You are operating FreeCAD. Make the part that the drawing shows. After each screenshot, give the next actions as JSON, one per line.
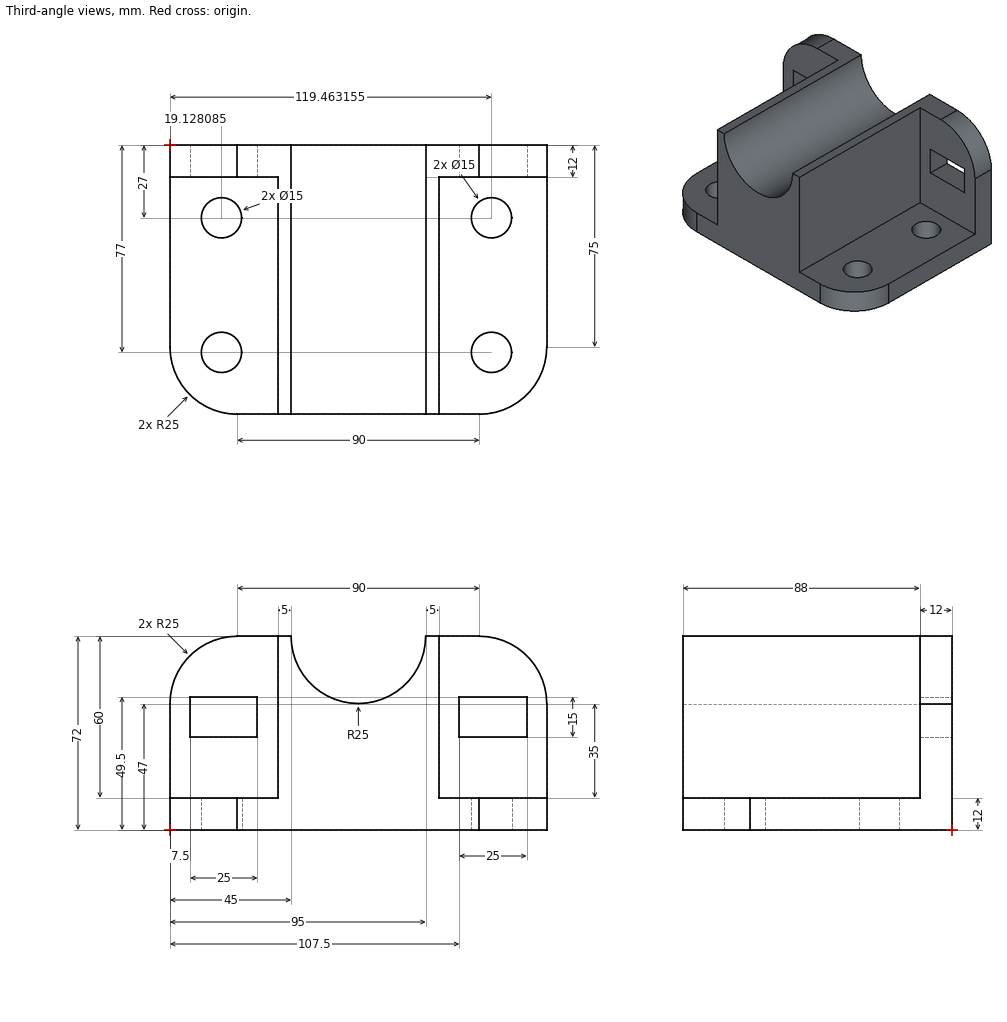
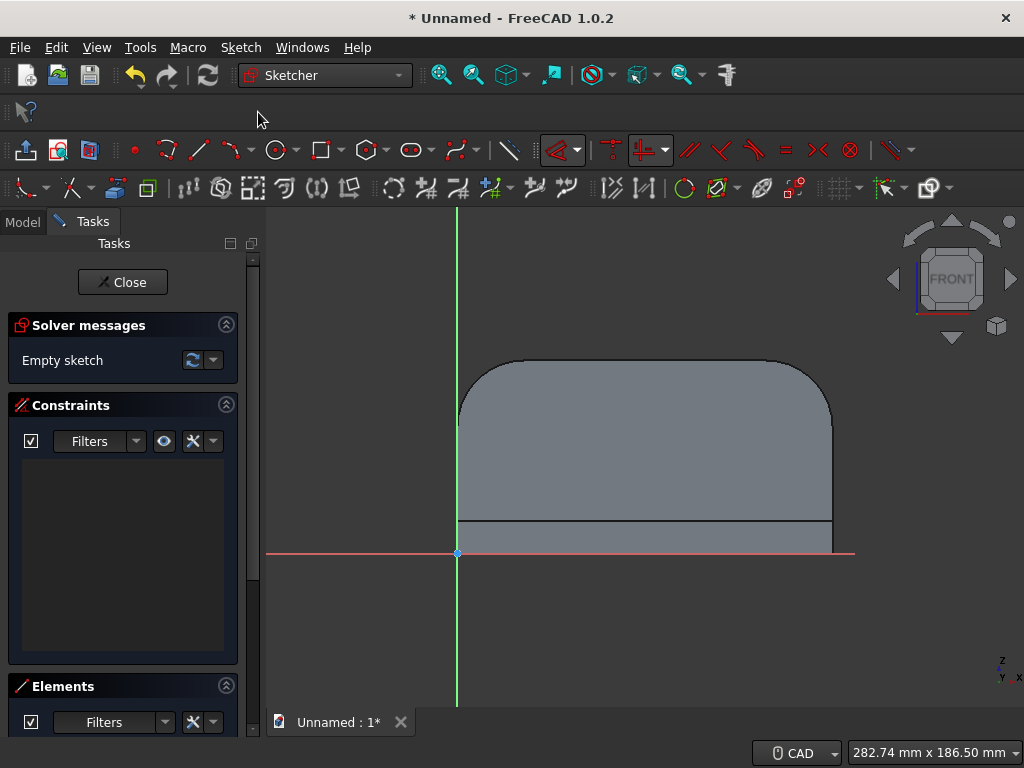
{"action": "scroll", "coordinate": [622, 457], "scroll_direction": "up", "scroll_amount": 2}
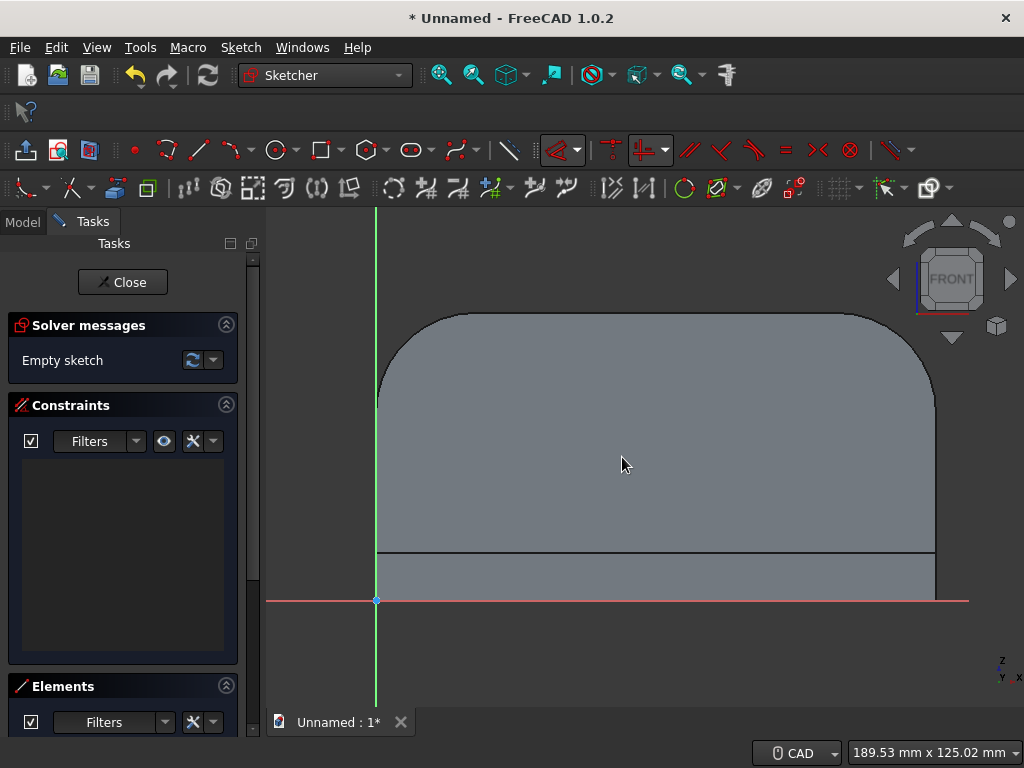
{"action": "left_click", "coordinate": [168, 150]}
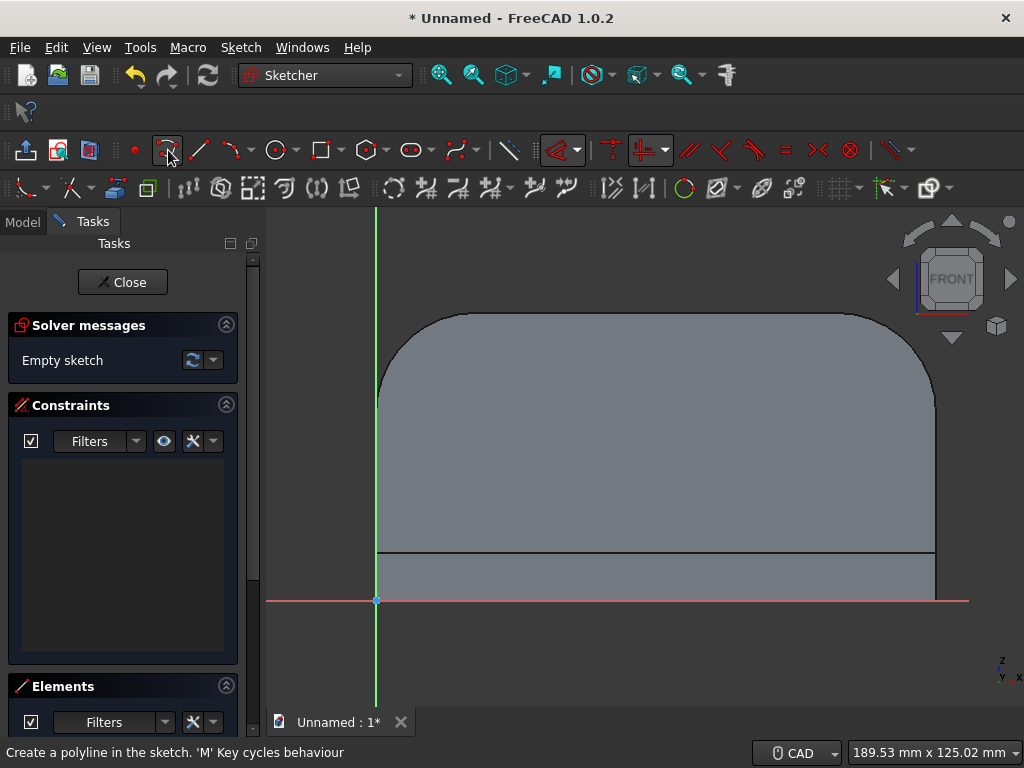
{"action": "left_click", "coordinate": [556, 313]}
{"action": "left_click", "coordinate": [536, 313]}
{"action": "left_click", "coordinate": [536, 553]}
{"action": "left_click", "coordinate": [776, 553]}
{"action": "left_click", "coordinate": [776, 313]}
{"action": "left_click", "coordinate": [756, 313]}
{"action": "right_click", "coordinate": [756, 313]}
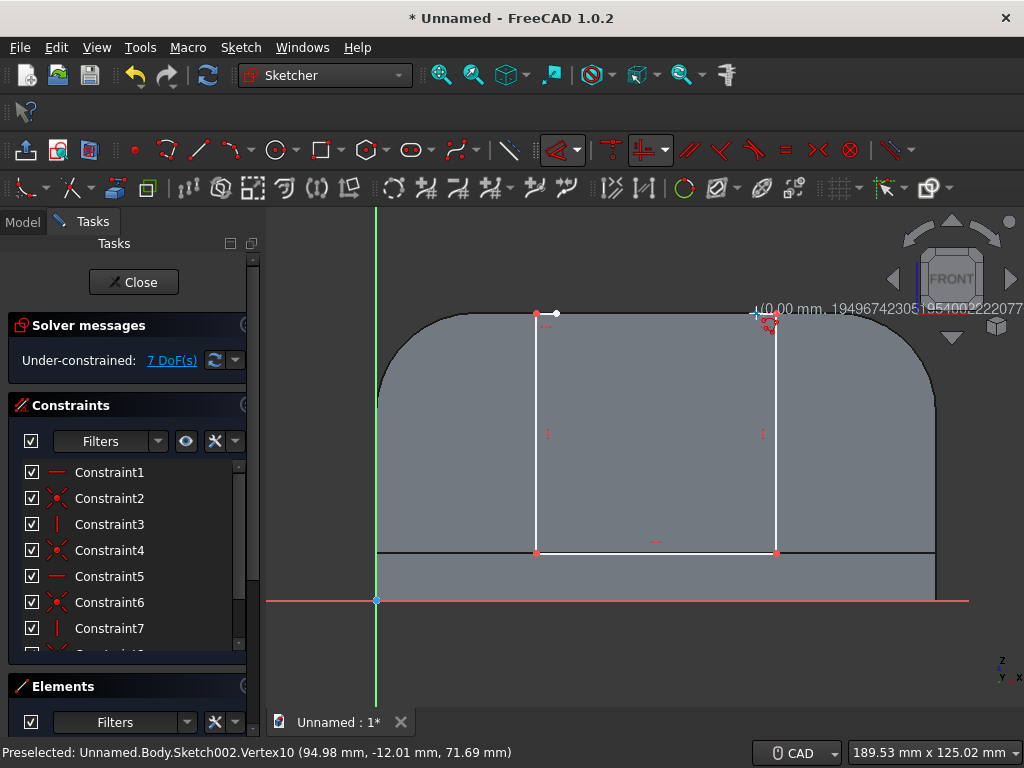
{"action": "left_click", "coordinate": [232, 150]}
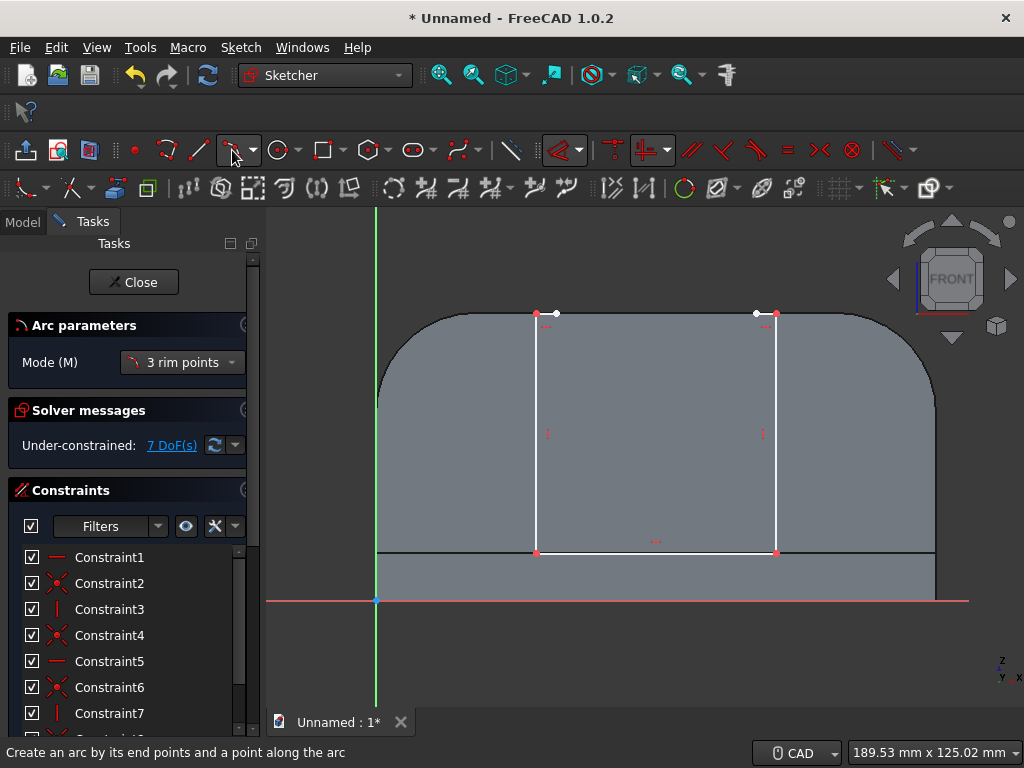
{"action": "scroll", "coordinate": [756, 313], "scroll_direction": "up", "scroll_amount": 3}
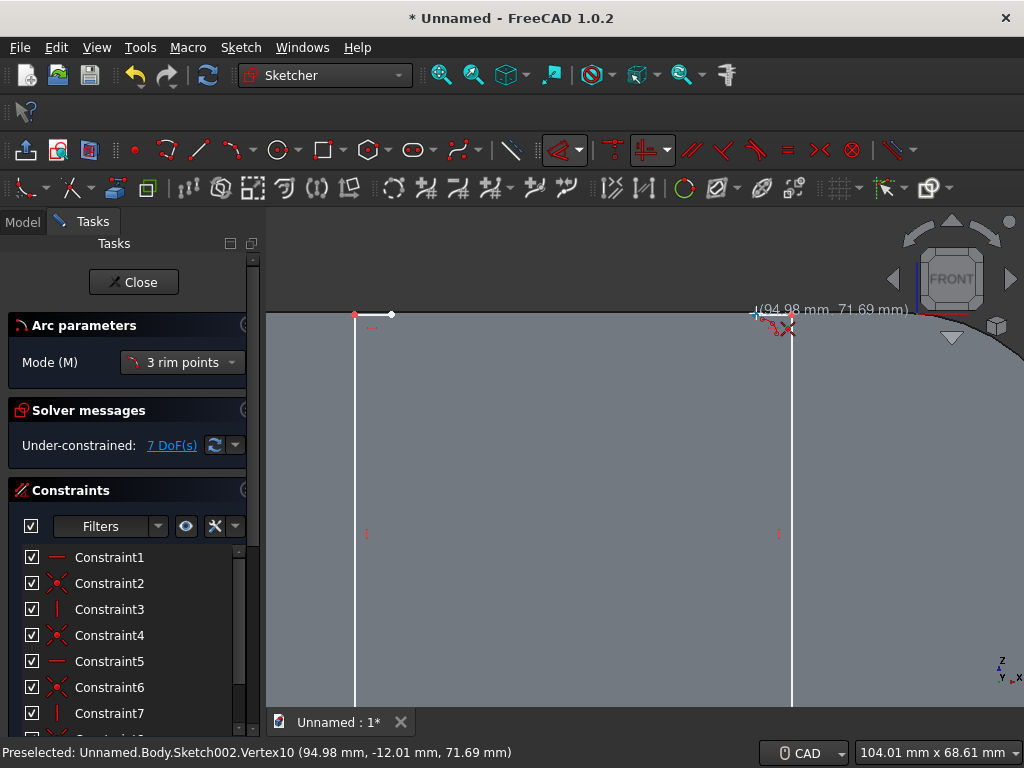
{"action": "left_click", "coordinate": [755, 315]}
{"action": "left_click", "coordinate": [391, 315]}
{"action": "left_click", "coordinate": [573, 495]}
{"action": "key", "text": "Escape"}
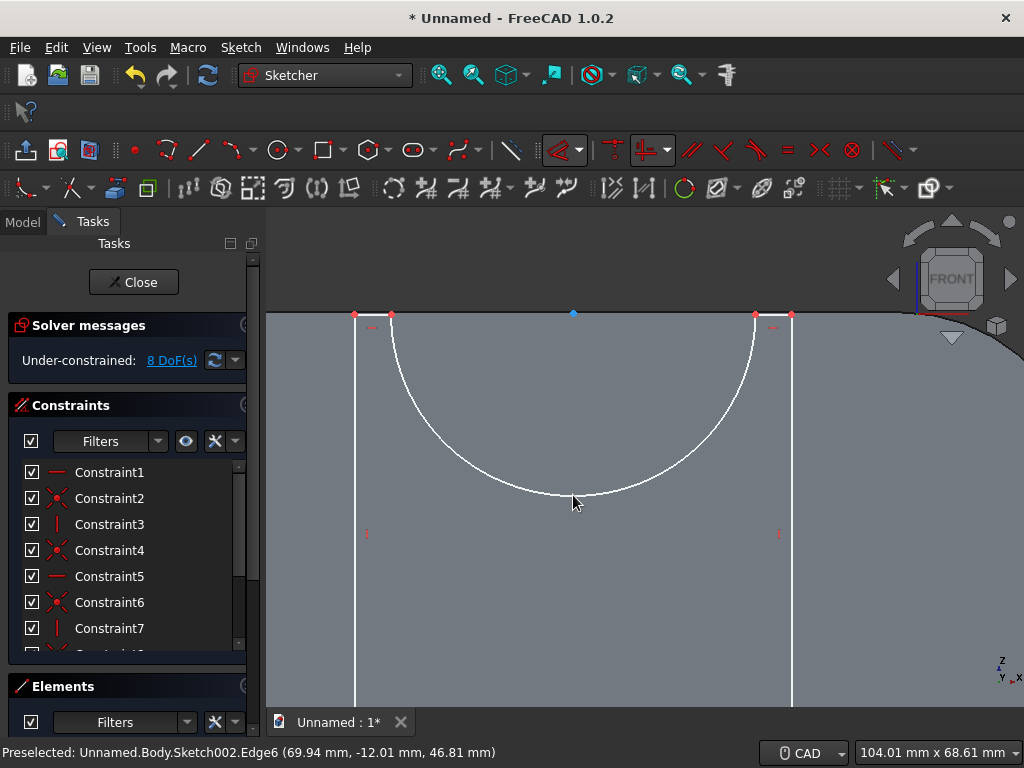
{"action": "left_click", "coordinate": [466, 461]}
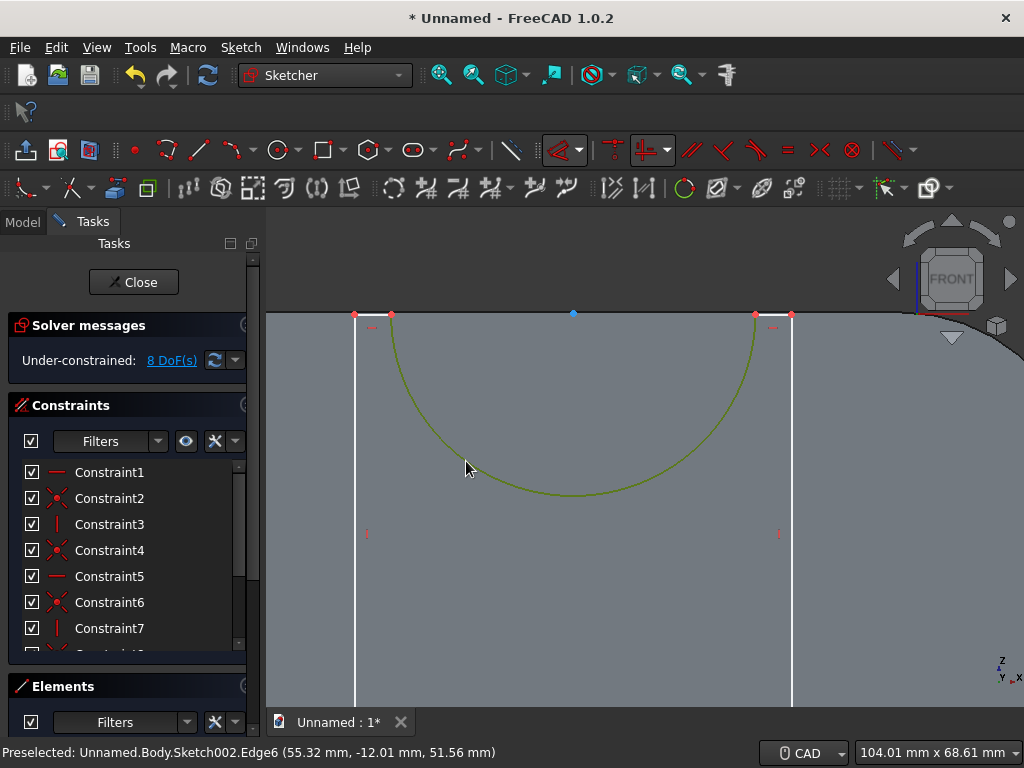
{"action": "key", "text": "k r"}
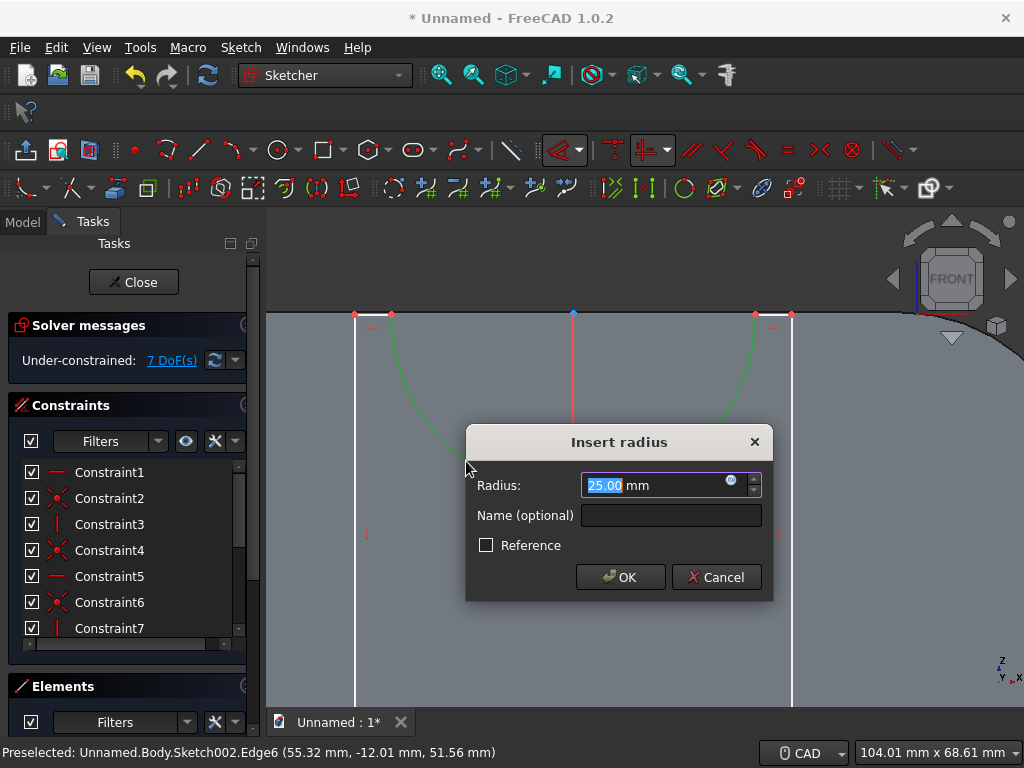
{"action": "type", "text": "25"}
{"action": "key", "text": "Return"}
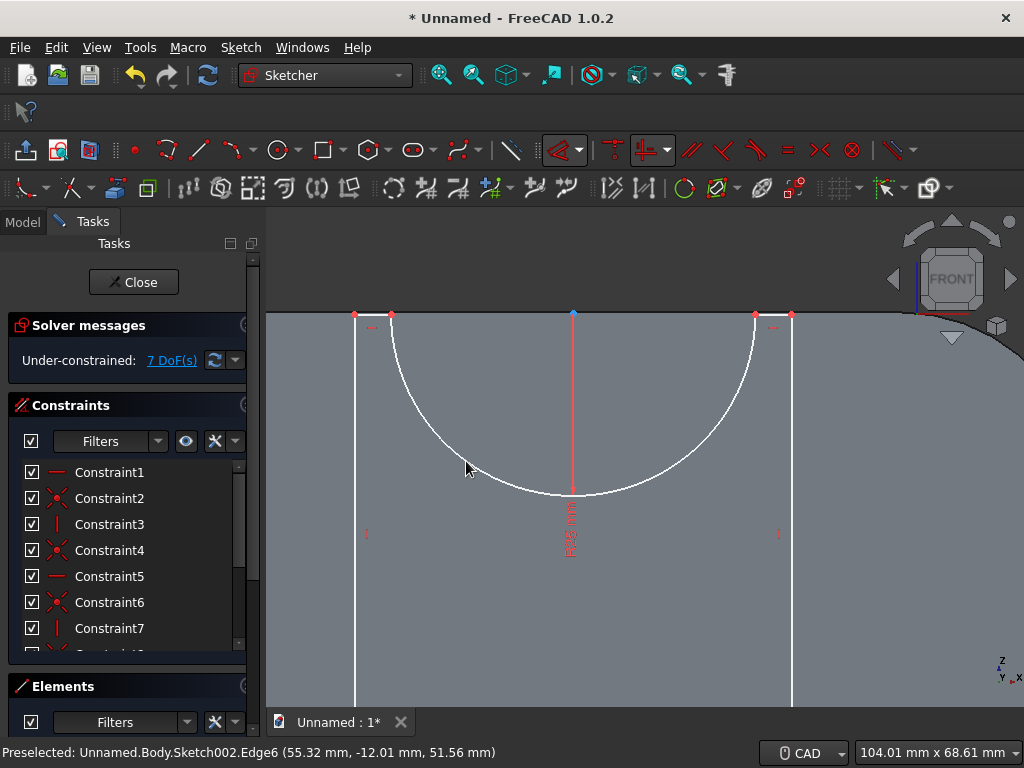
{"action": "scroll", "coordinate": [380, 315], "scroll_direction": "up", "scroll_amount": 2}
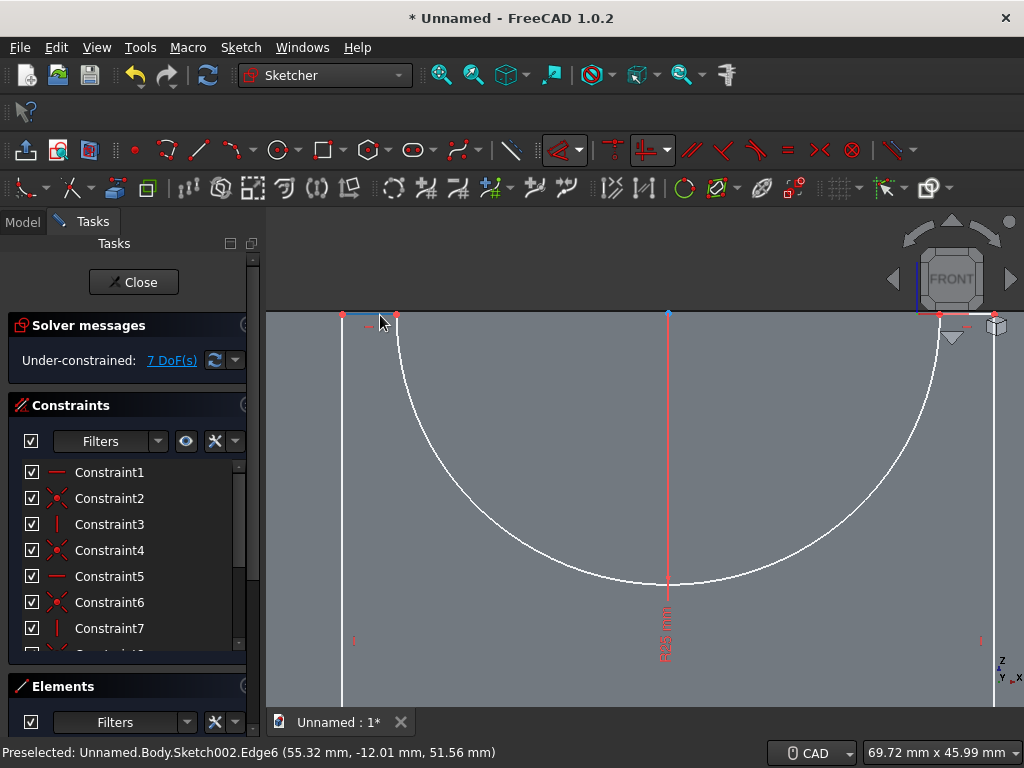
{"action": "left_click", "coordinate": [380, 314]}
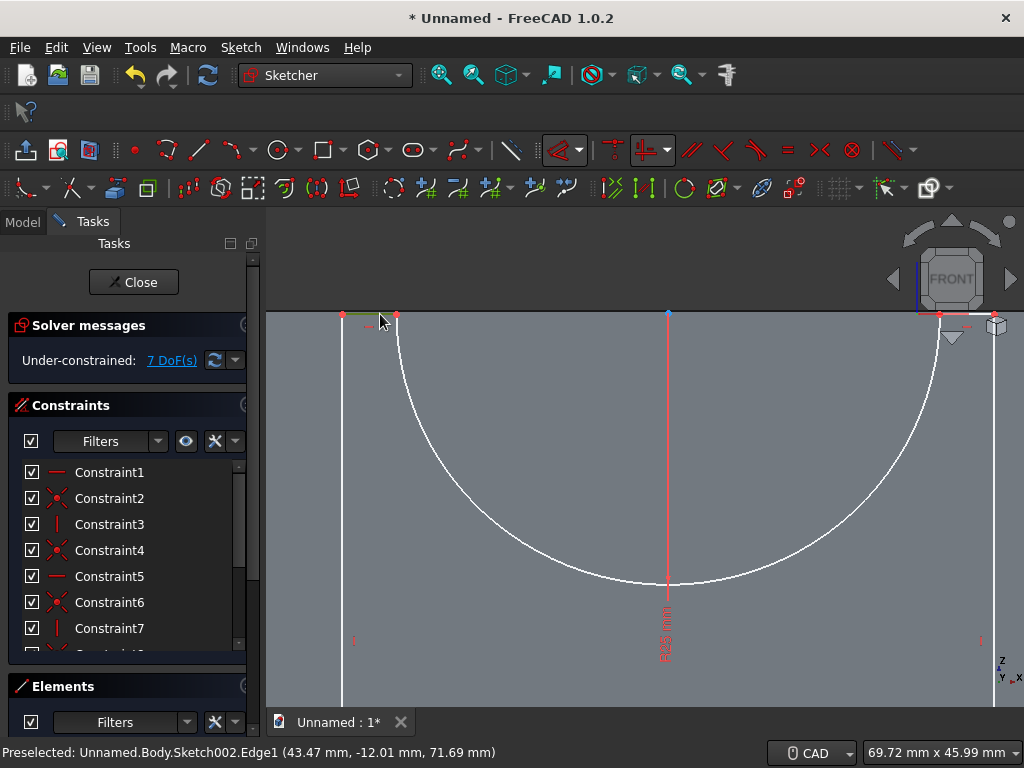
{"action": "key", "text": "l"}